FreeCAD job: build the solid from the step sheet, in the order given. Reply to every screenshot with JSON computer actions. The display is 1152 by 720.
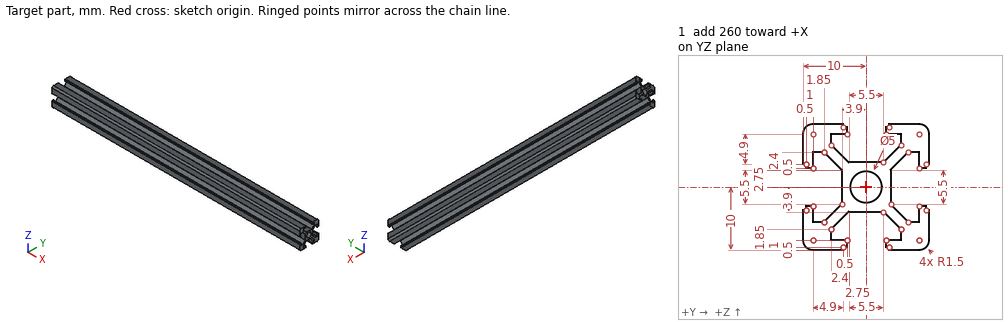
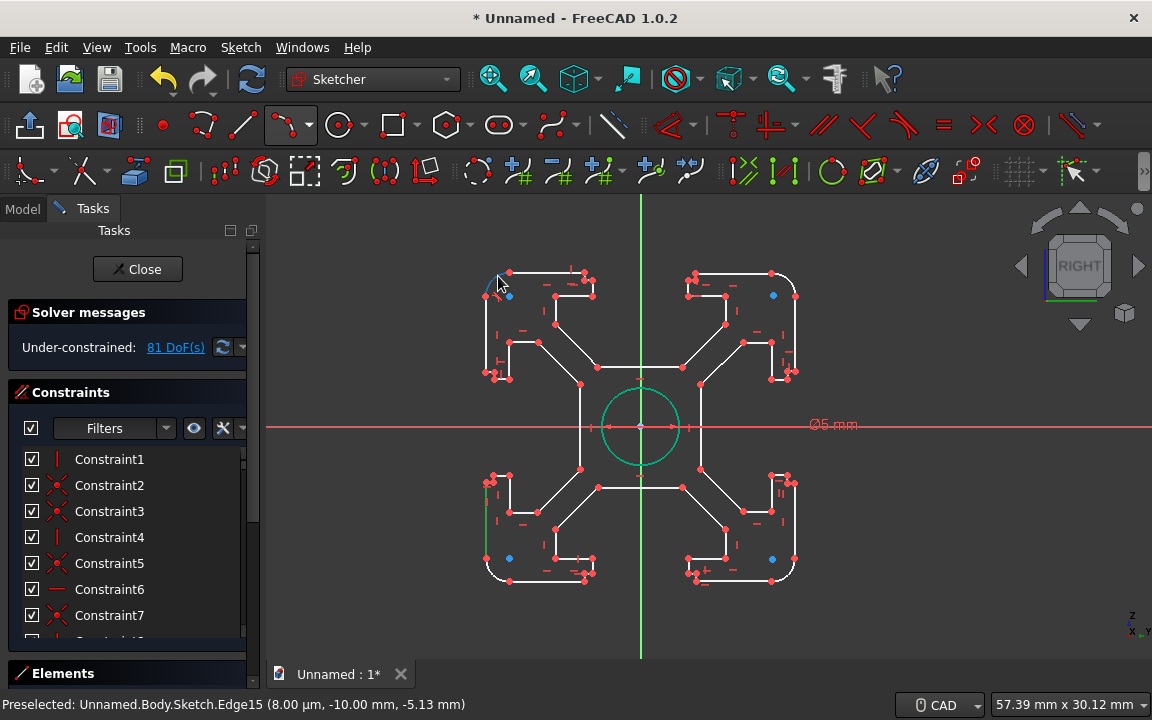
{"action": "scroll", "coordinate": [489, 569], "scroll_direction": "up", "scroll_amount": 2}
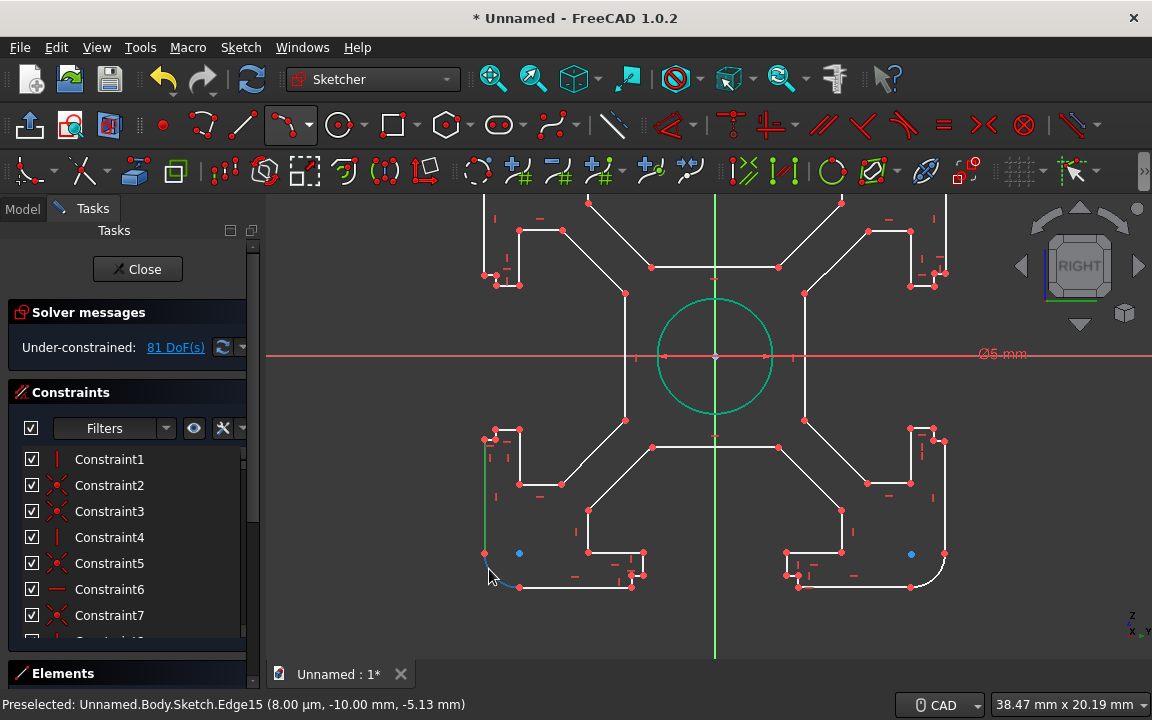
{"action": "left_click", "coordinate": [489, 569]}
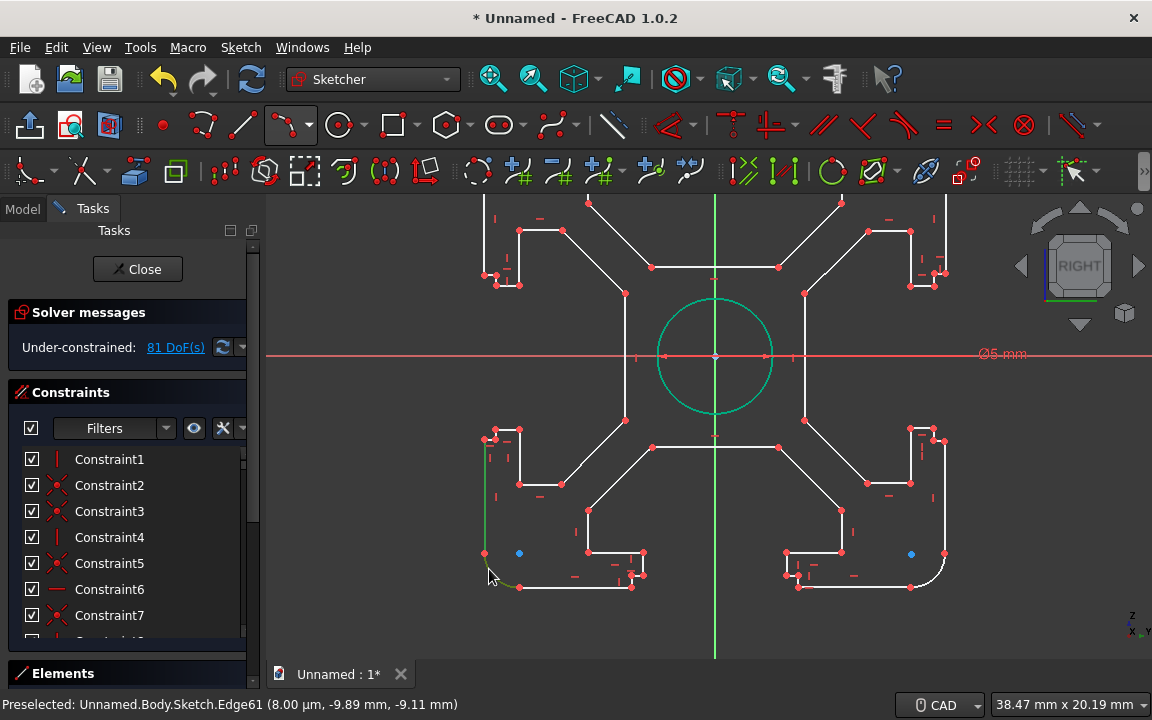
{"action": "key", "text": "t"}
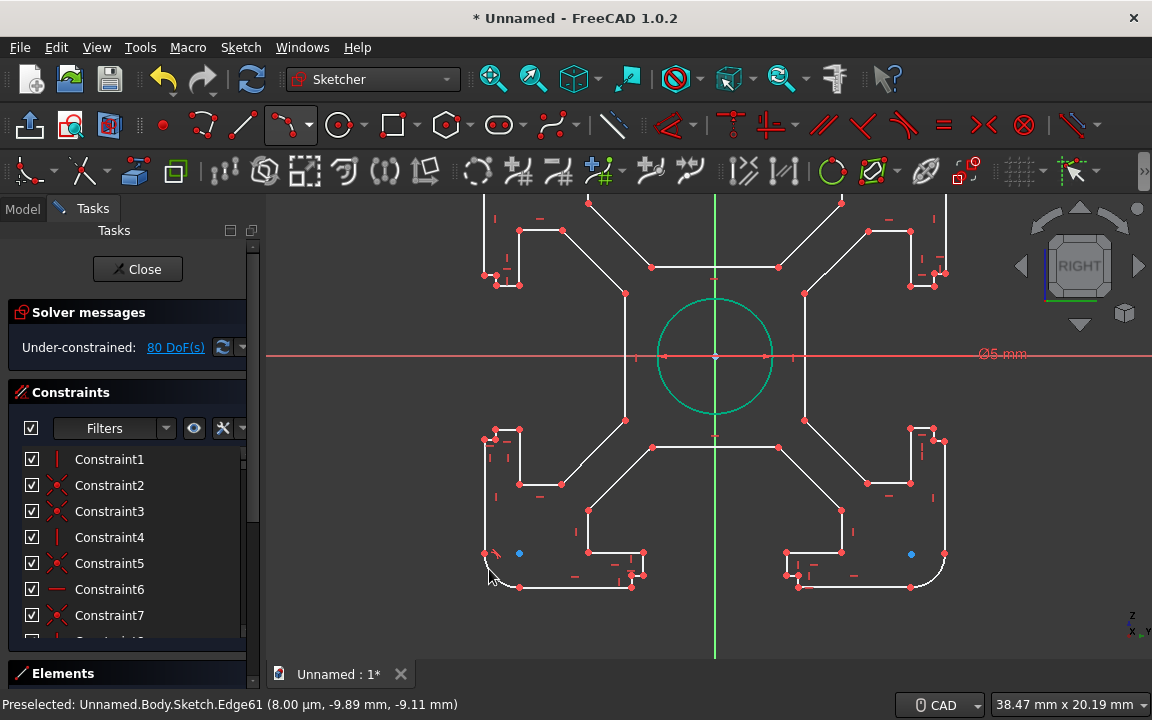
{"action": "left_click", "coordinate": [553, 588]}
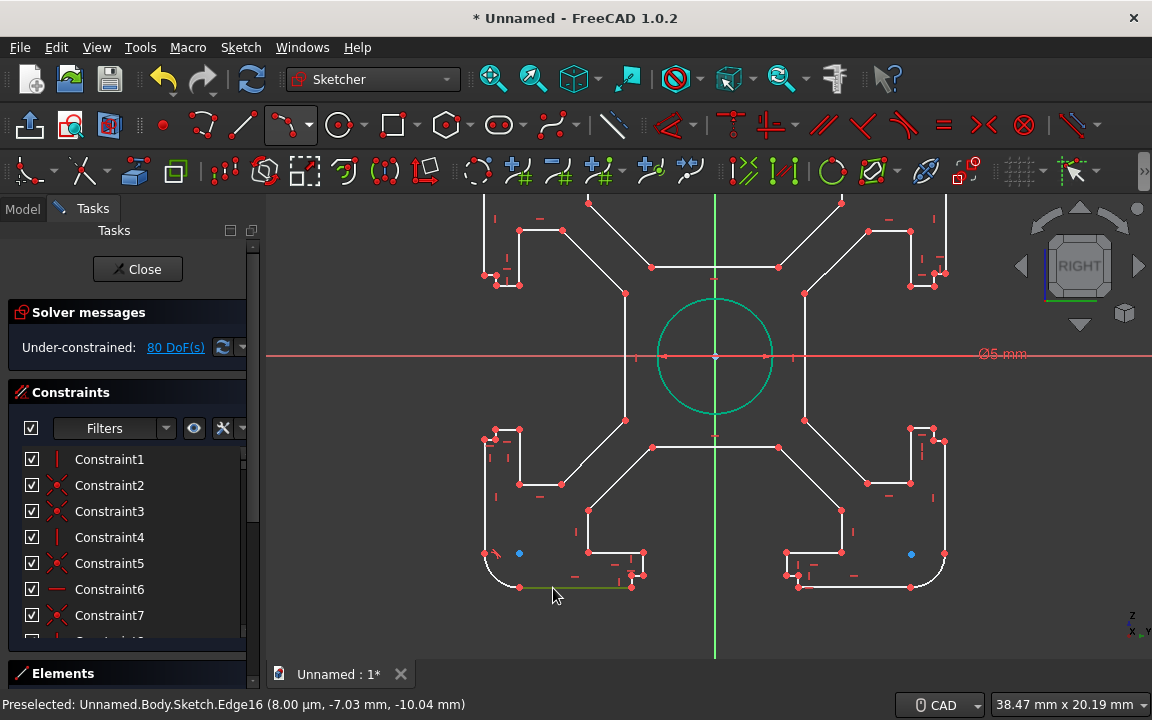
{"action": "left_click", "coordinate": [488, 569]}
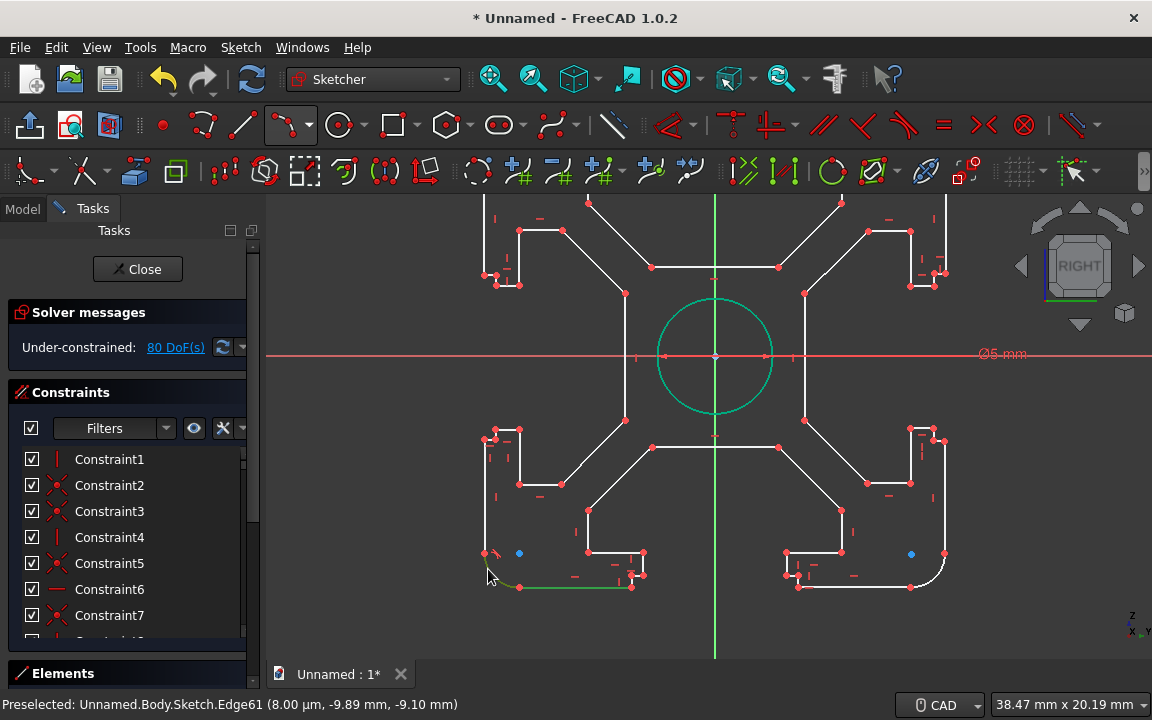
{"action": "key", "text": "t"}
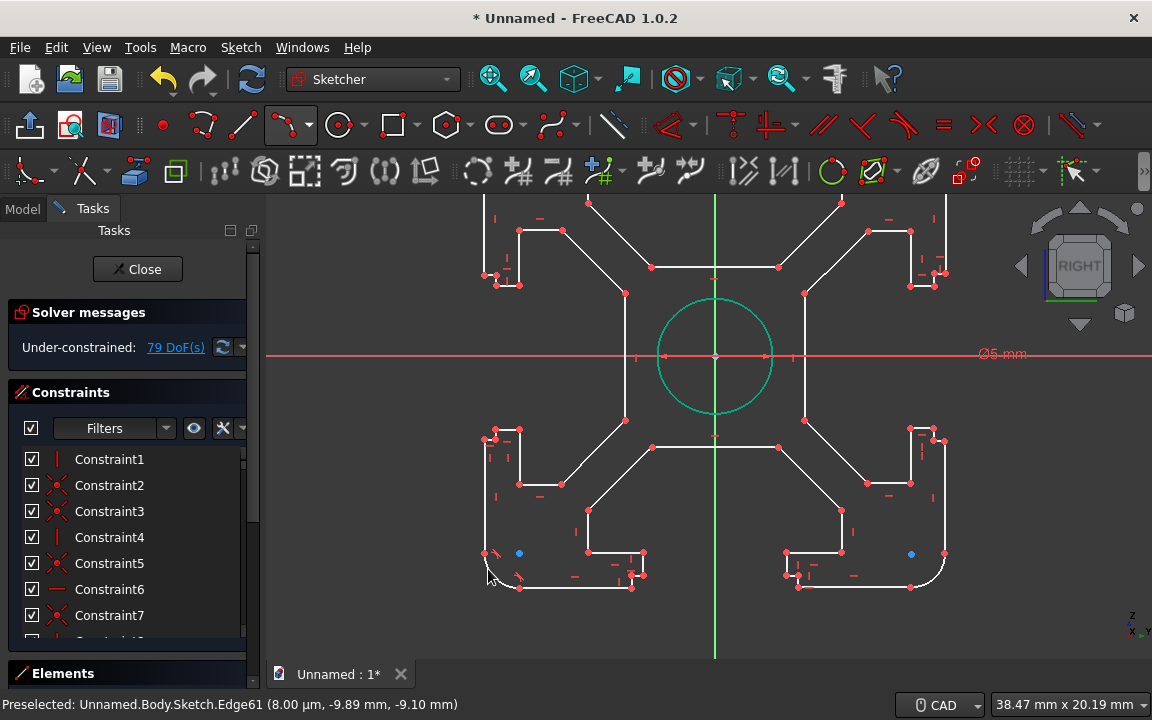
{"action": "left_click", "coordinate": [832, 587]}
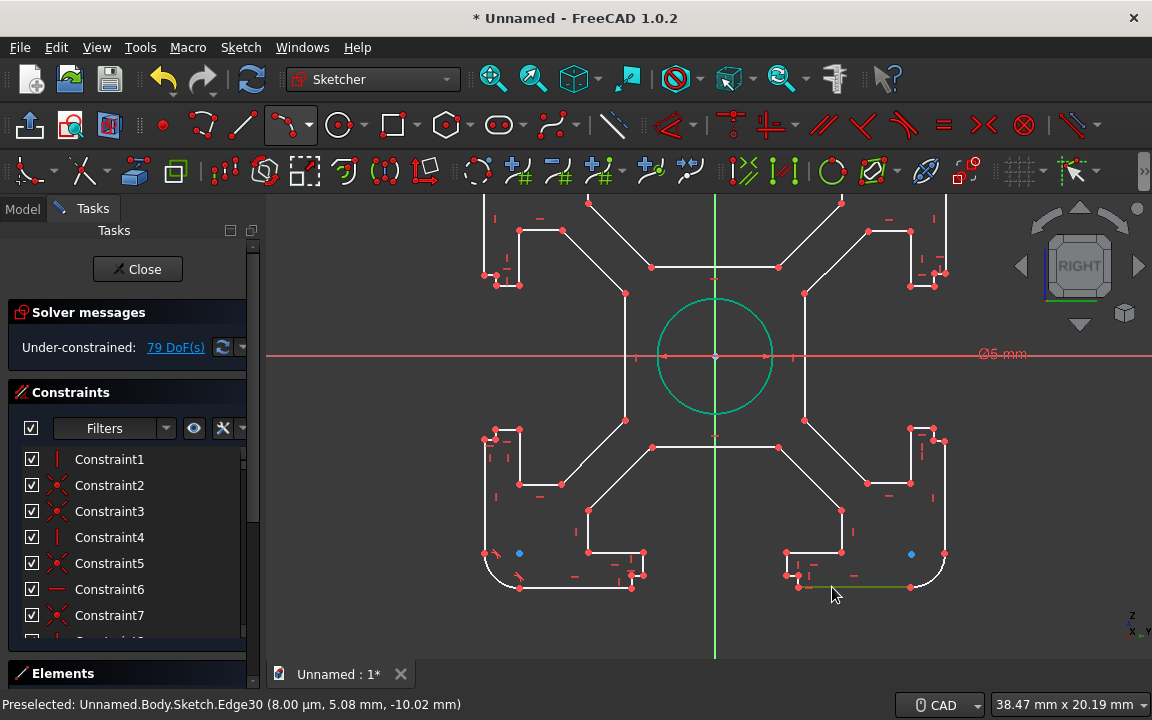
{"action": "left_click", "coordinate": [926, 584]}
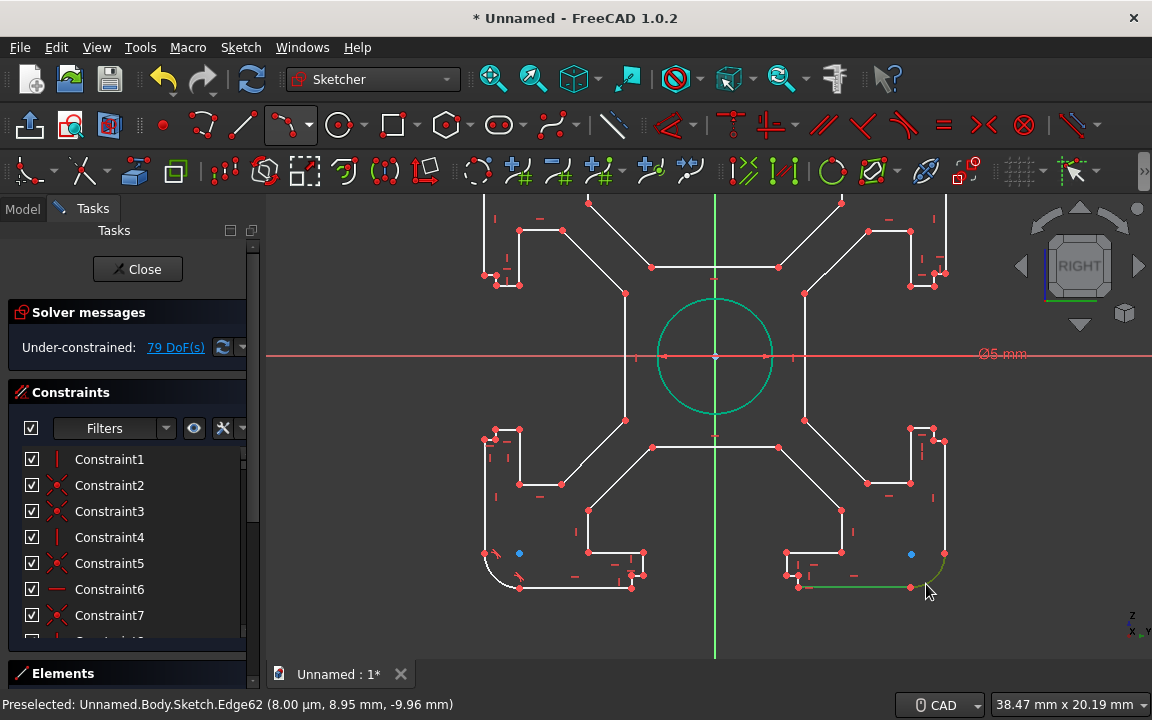
{"action": "left_click", "coordinate": [904, 126]}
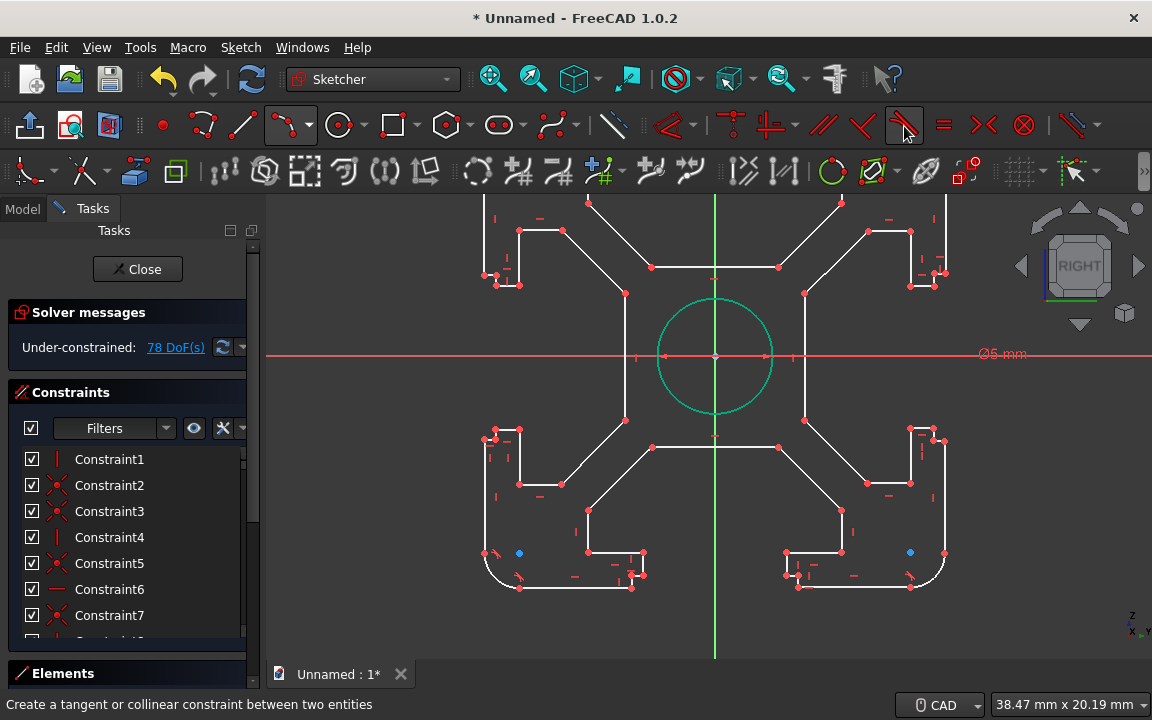
{"action": "left_click", "coordinate": [945, 520]}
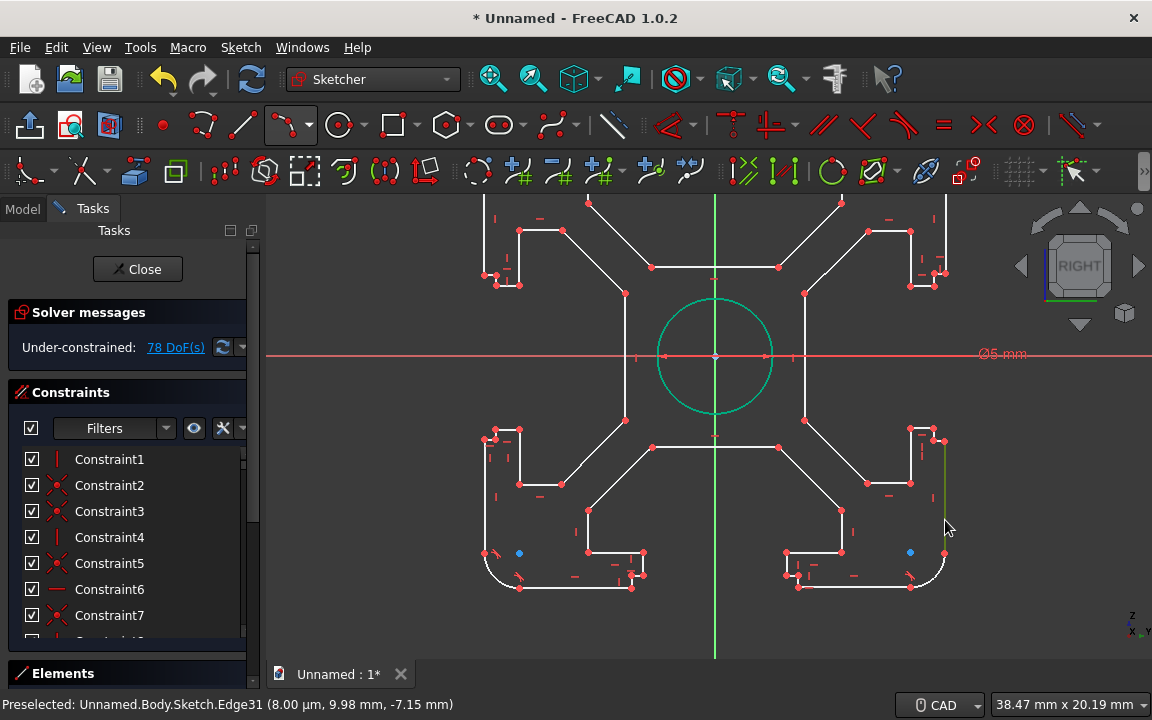
{"action": "left_click", "coordinate": [926, 584]}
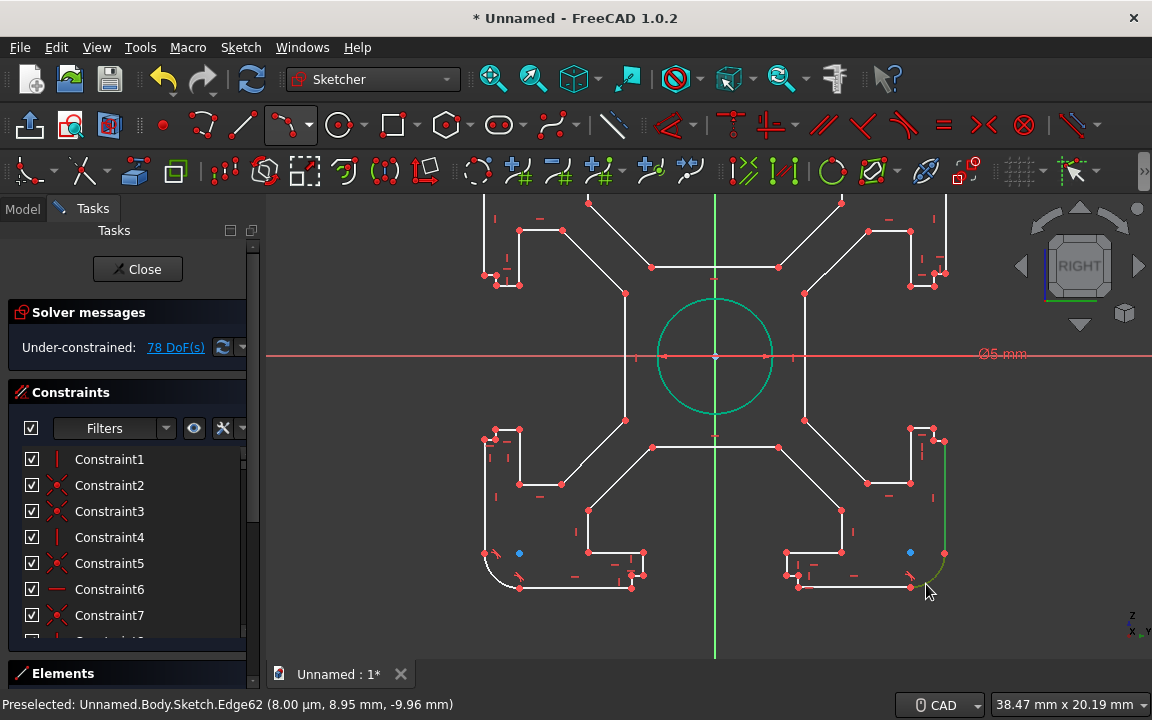
{"action": "key", "text": "t"}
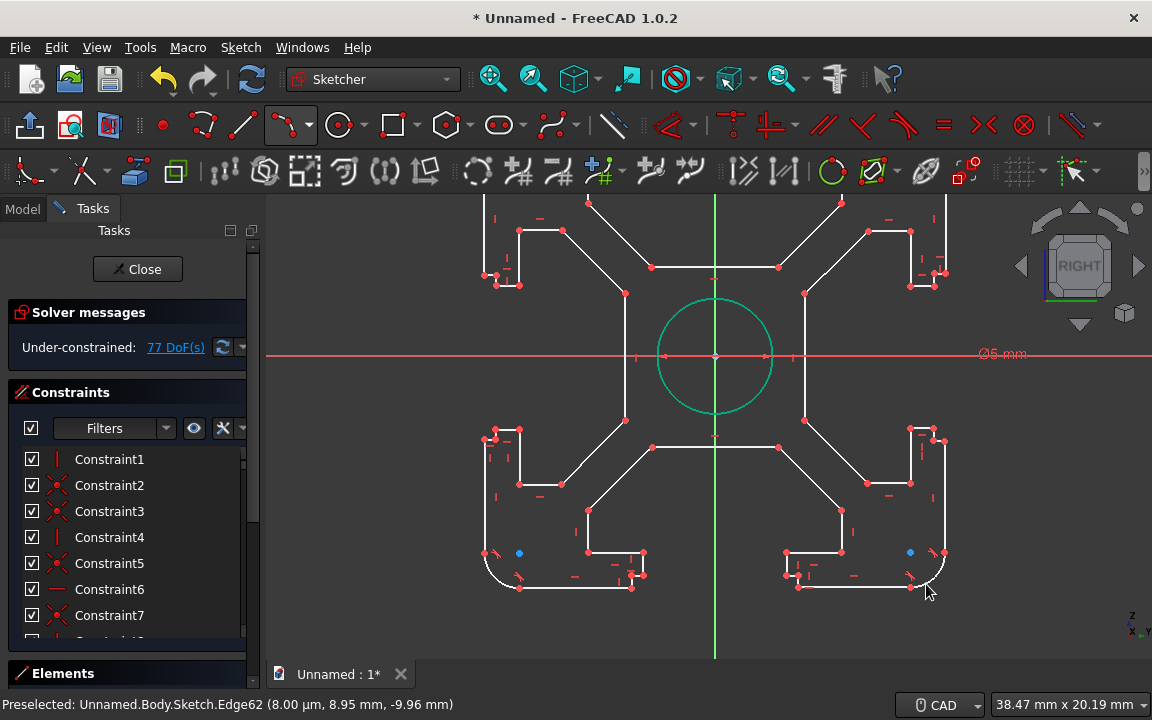
{"action": "left_click", "coordinate": [946, 240]}